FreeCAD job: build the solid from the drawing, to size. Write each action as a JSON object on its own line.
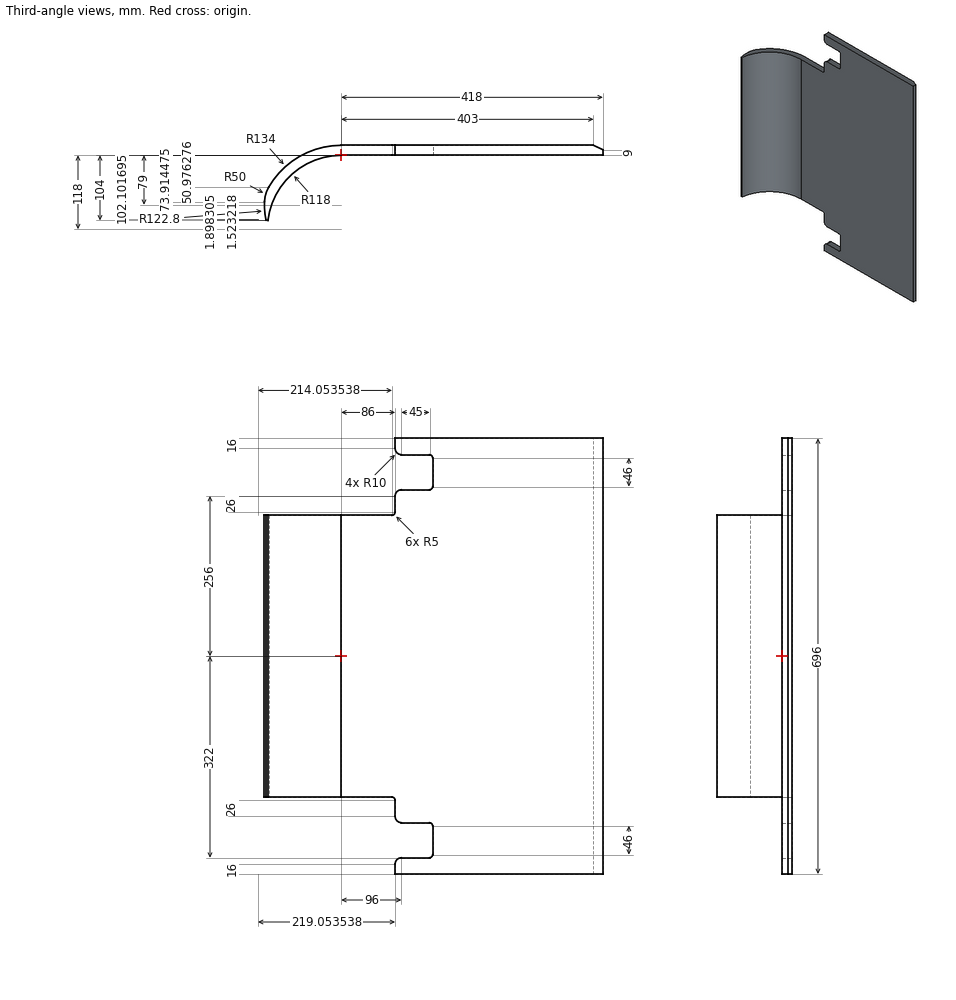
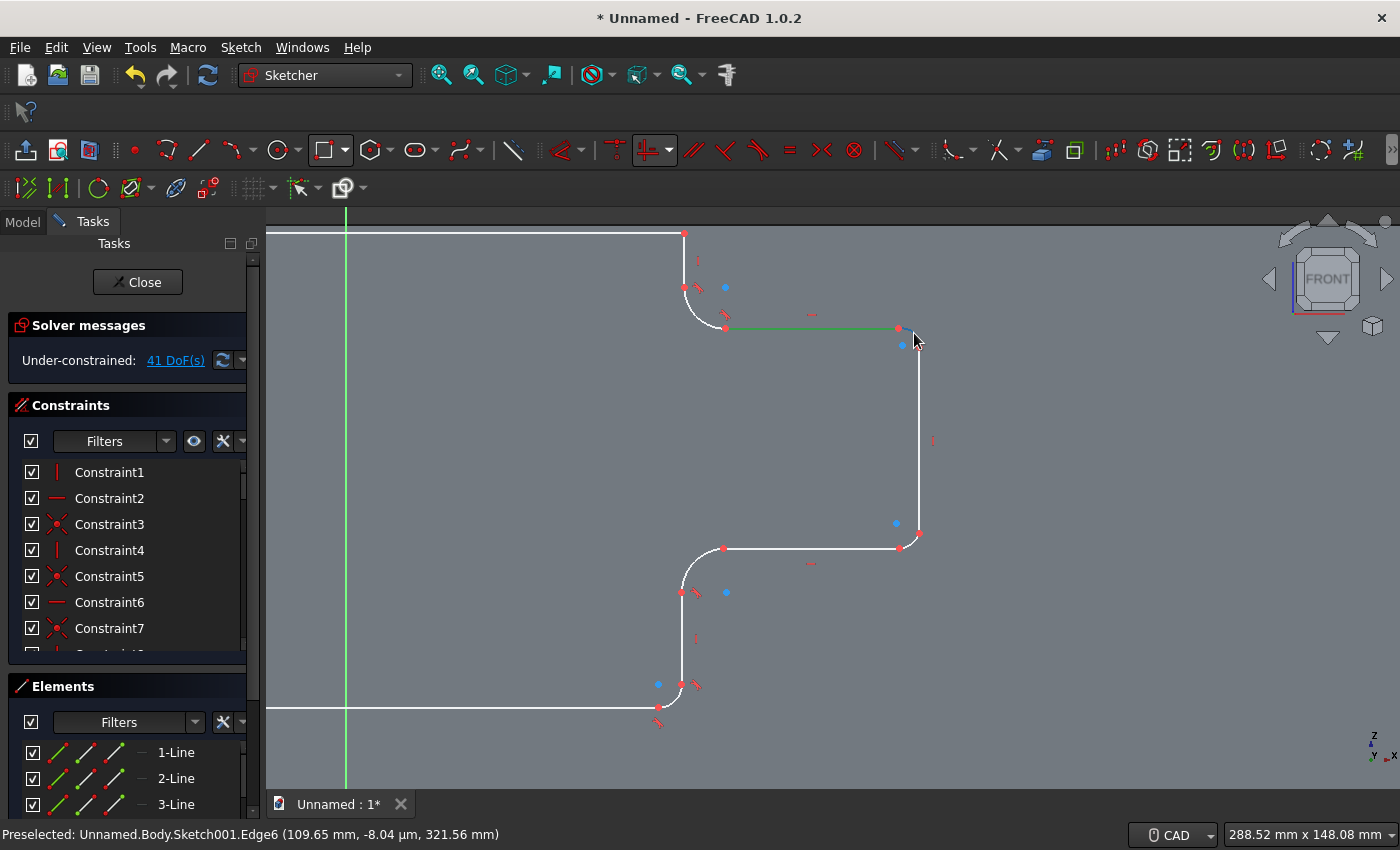
{"action": "left_click", "coordinate": [914, 333]}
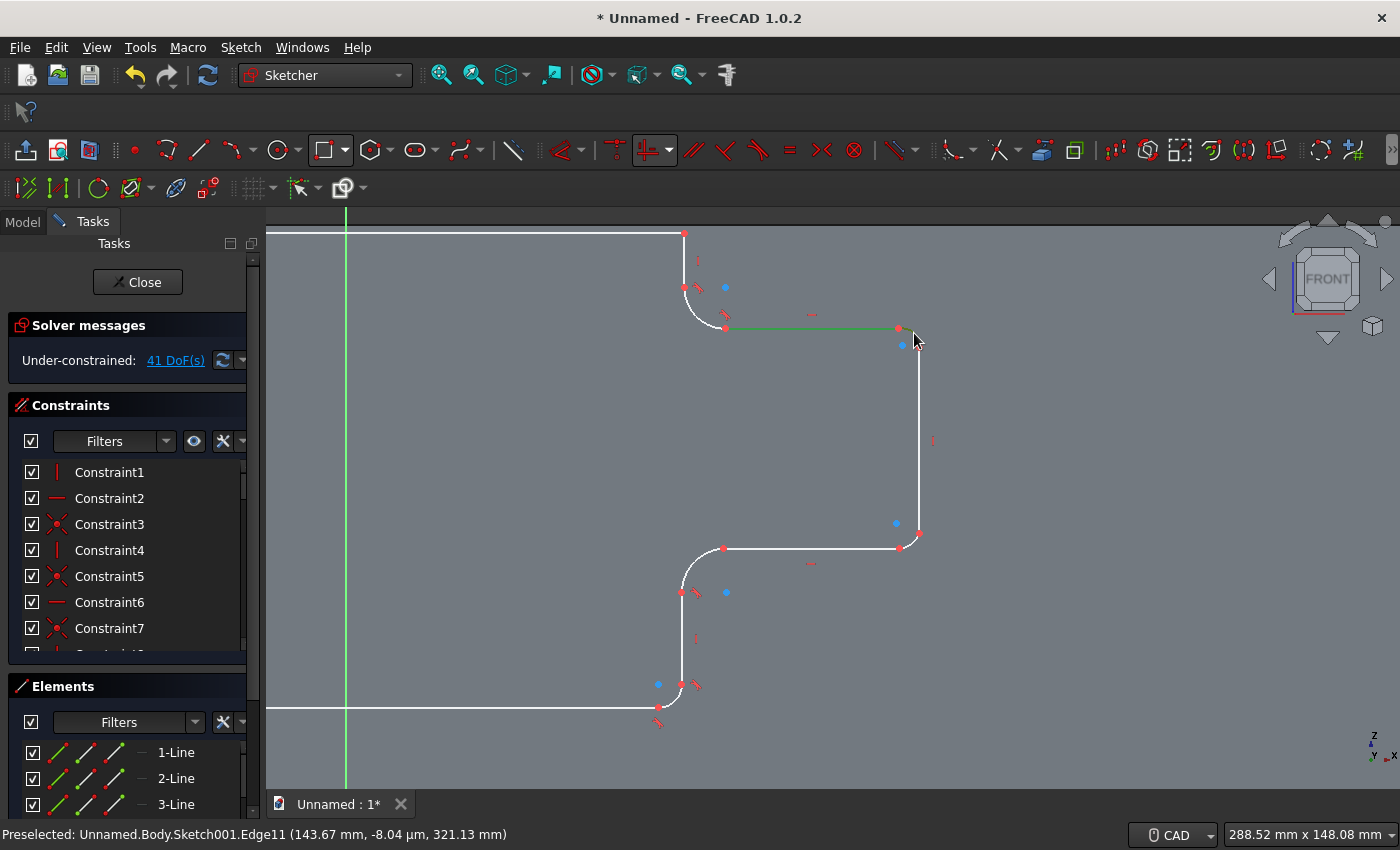
{"action": "left_click", "coordinate": [758, 150]}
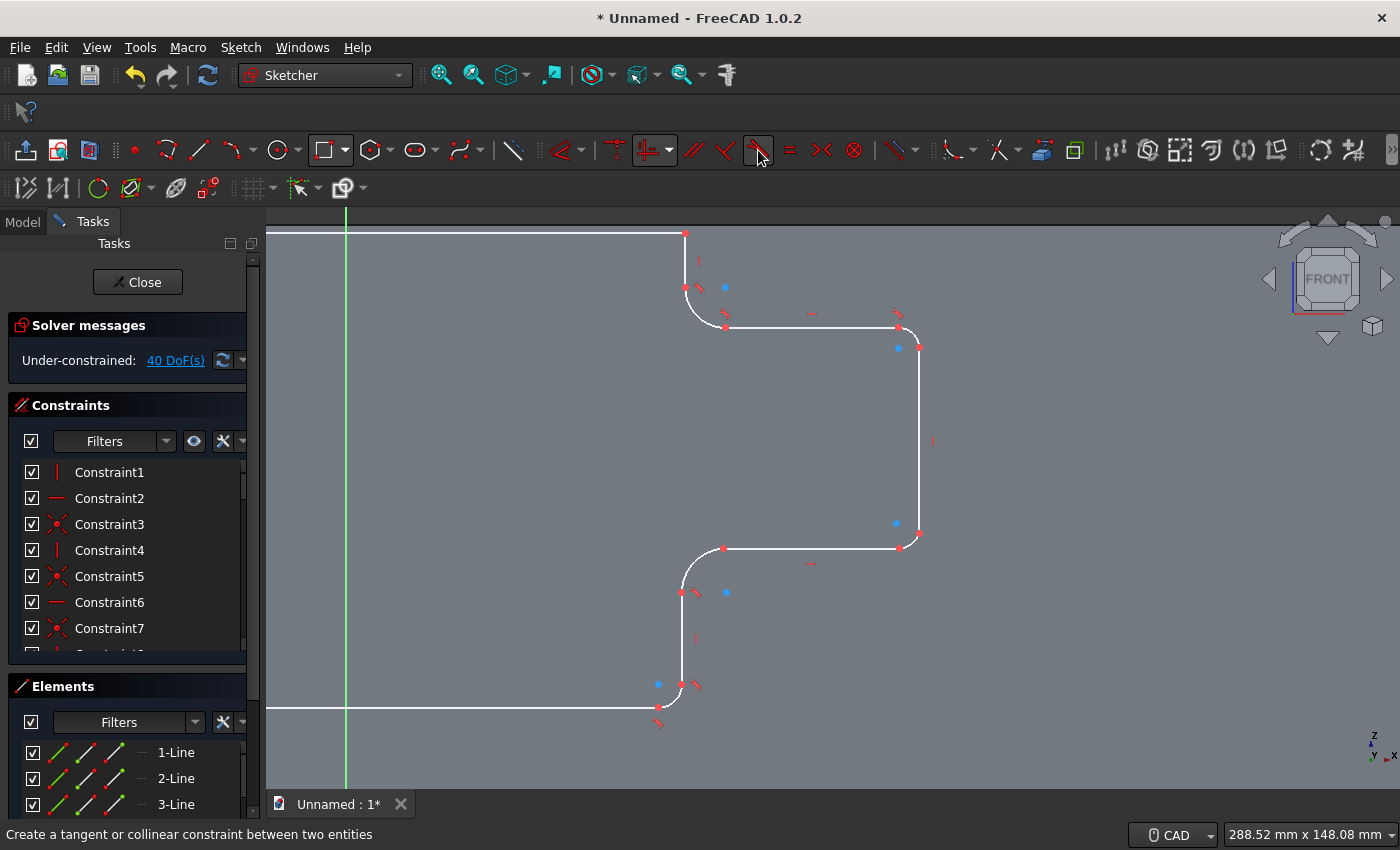
{"action": "scroll", "coordinate": [826, 327], "scroll_direction": "down", "scroll_amount": 10}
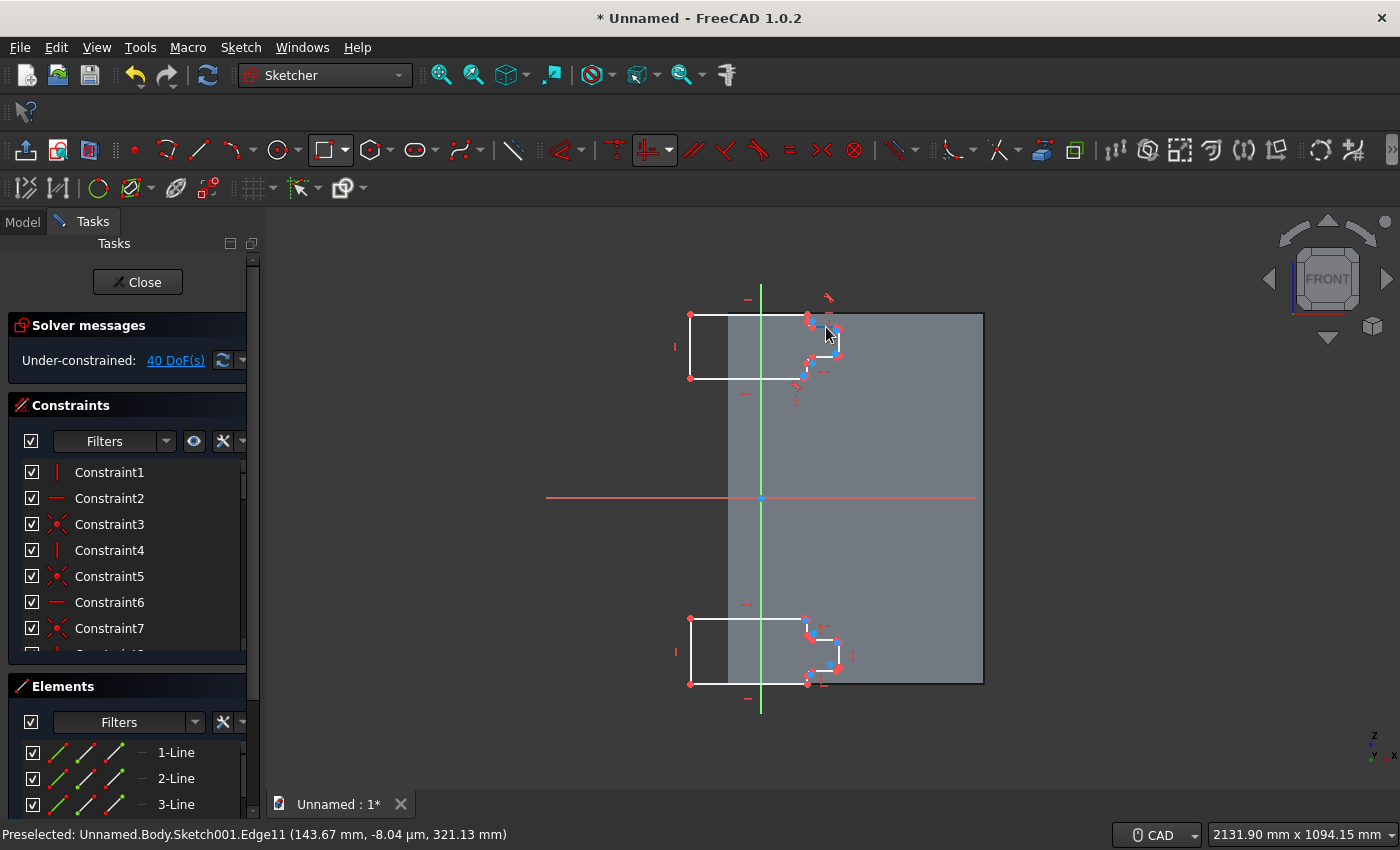
{"action": "scroll", "coordinate": [839, 338], "scroll_direction": "up", "scroll_amount": 4}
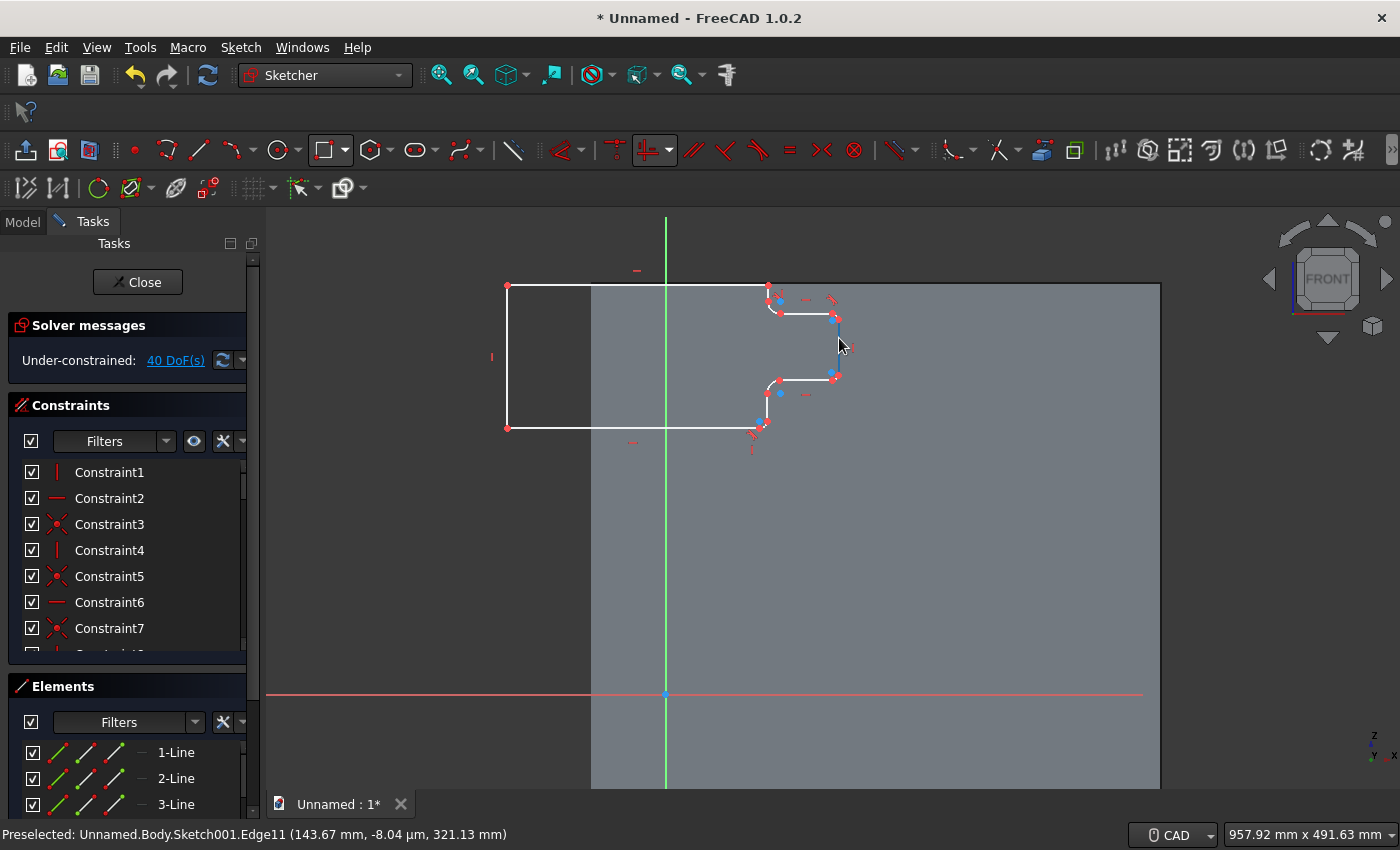
{"action": "left_click", "coordinate": [839, 337]}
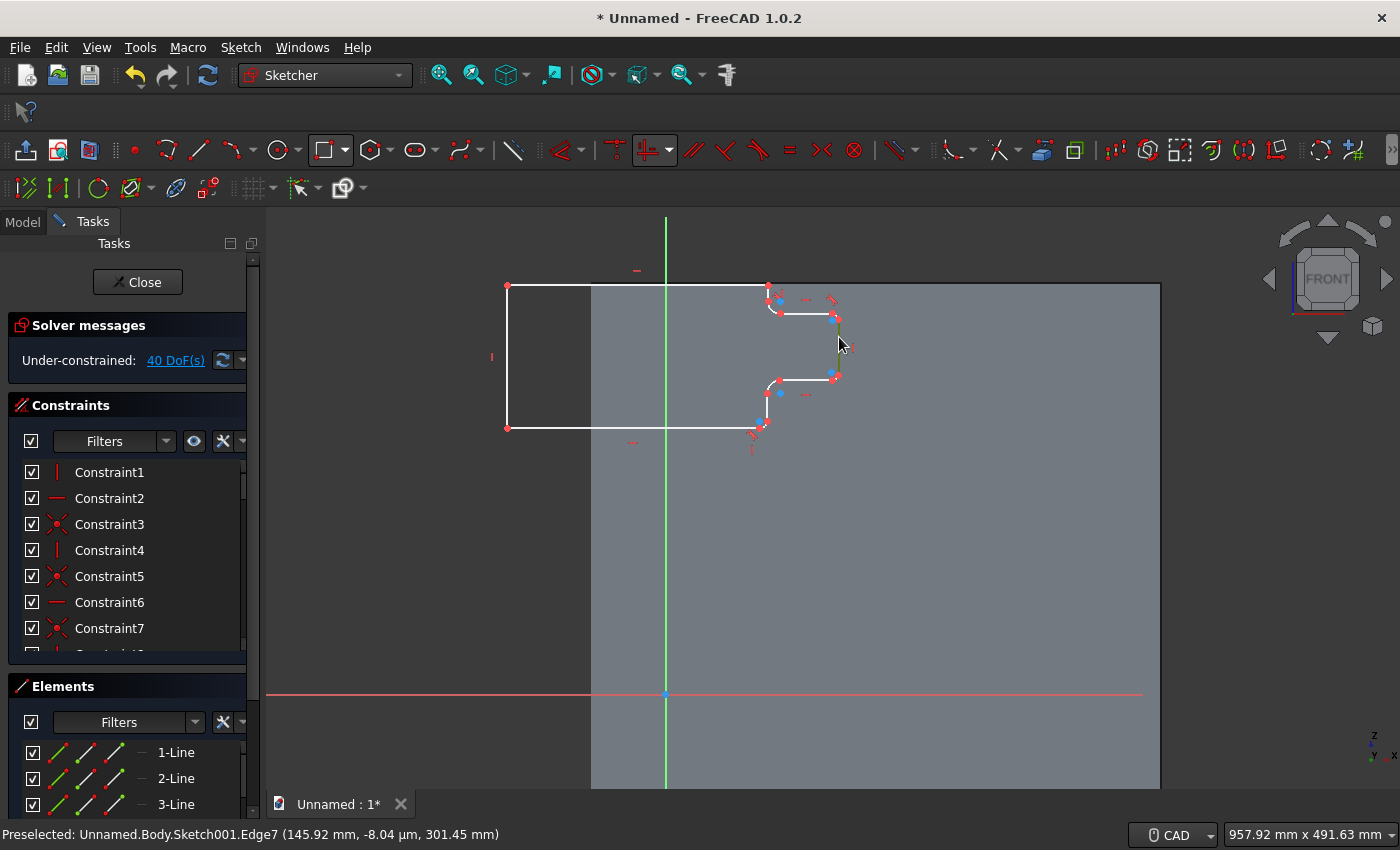
{"action": "scroll", "coordinate": [837, 316], "scroll_direction": "up", "scroll_amount": 6}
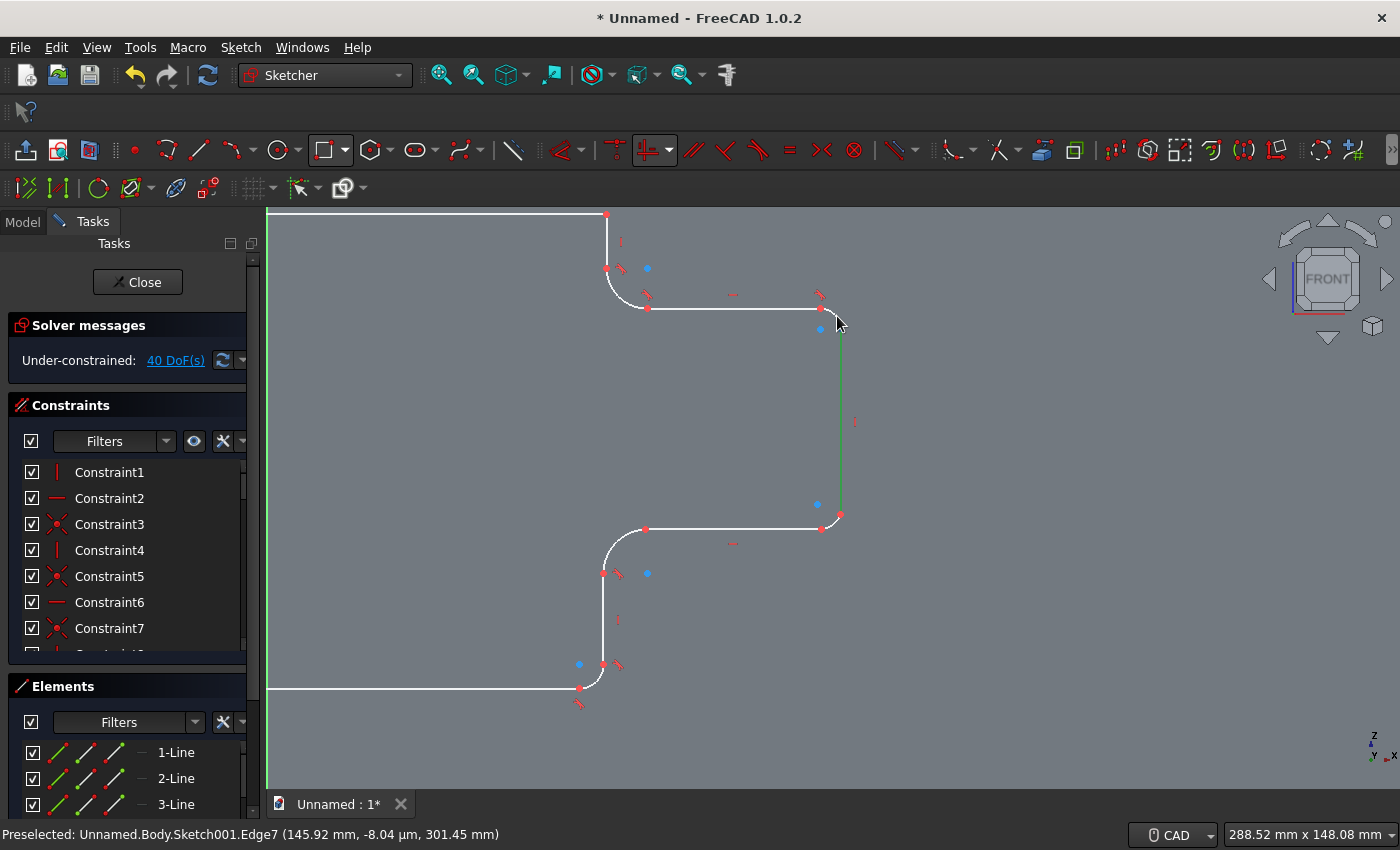
{"action": "left_click", "coordinate": [834, 314]}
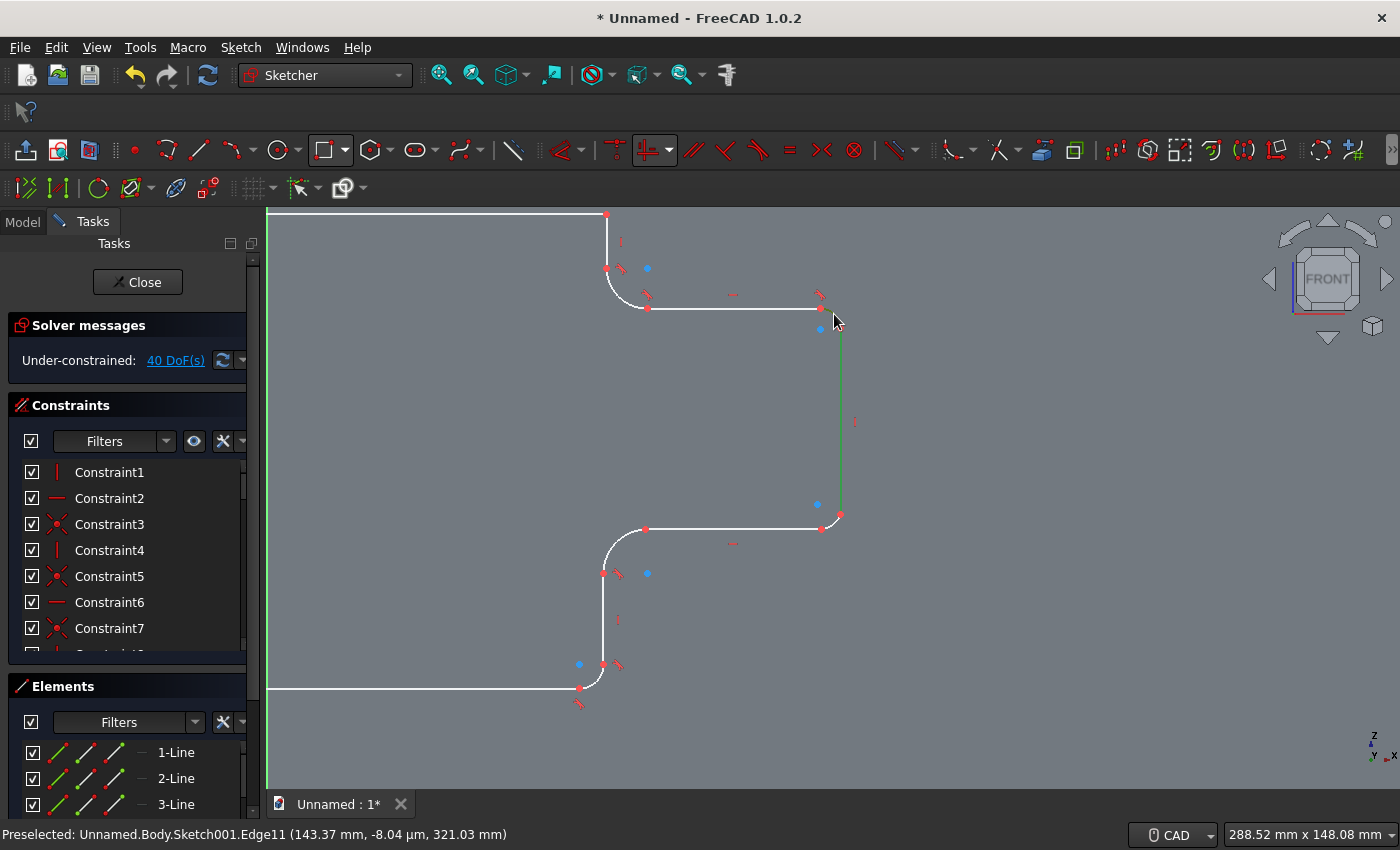
{"action": "left_click", "coordinate": [758, 150]}